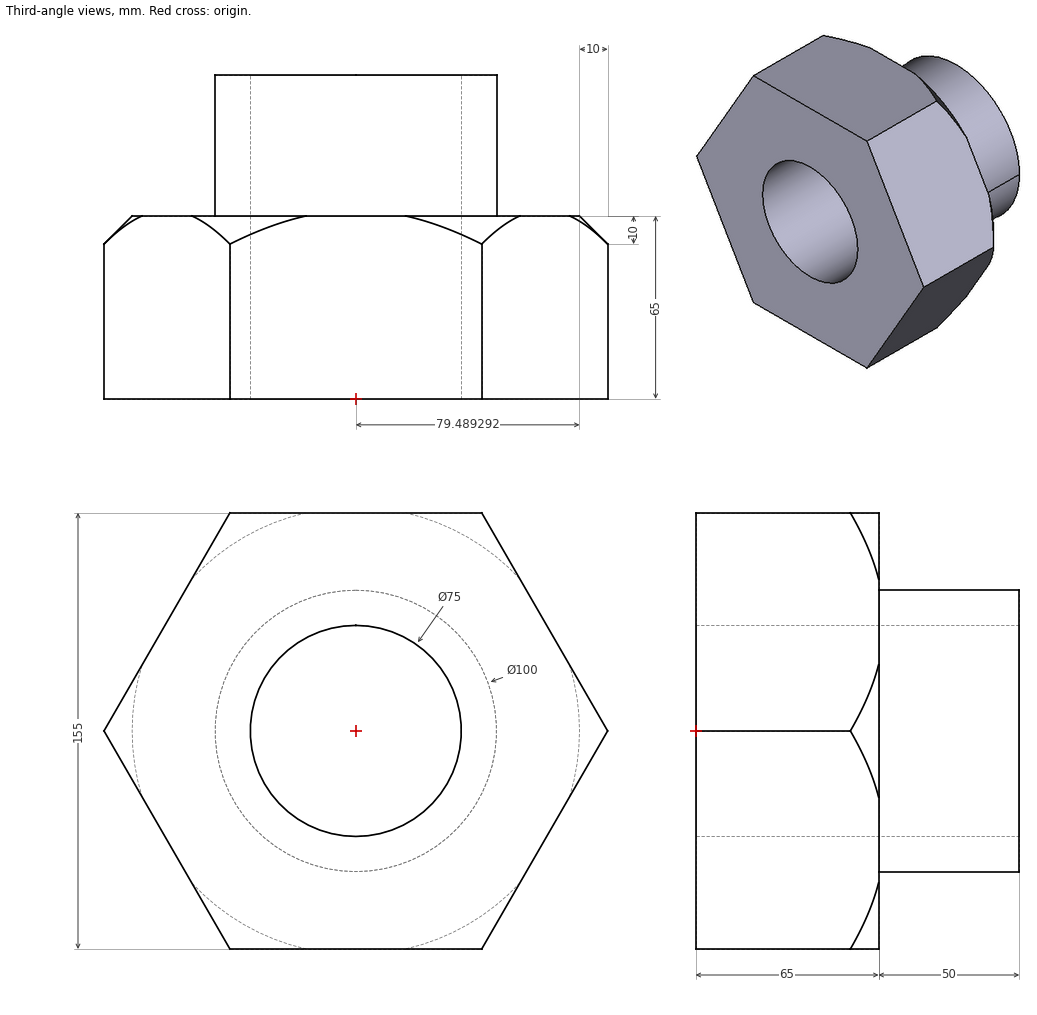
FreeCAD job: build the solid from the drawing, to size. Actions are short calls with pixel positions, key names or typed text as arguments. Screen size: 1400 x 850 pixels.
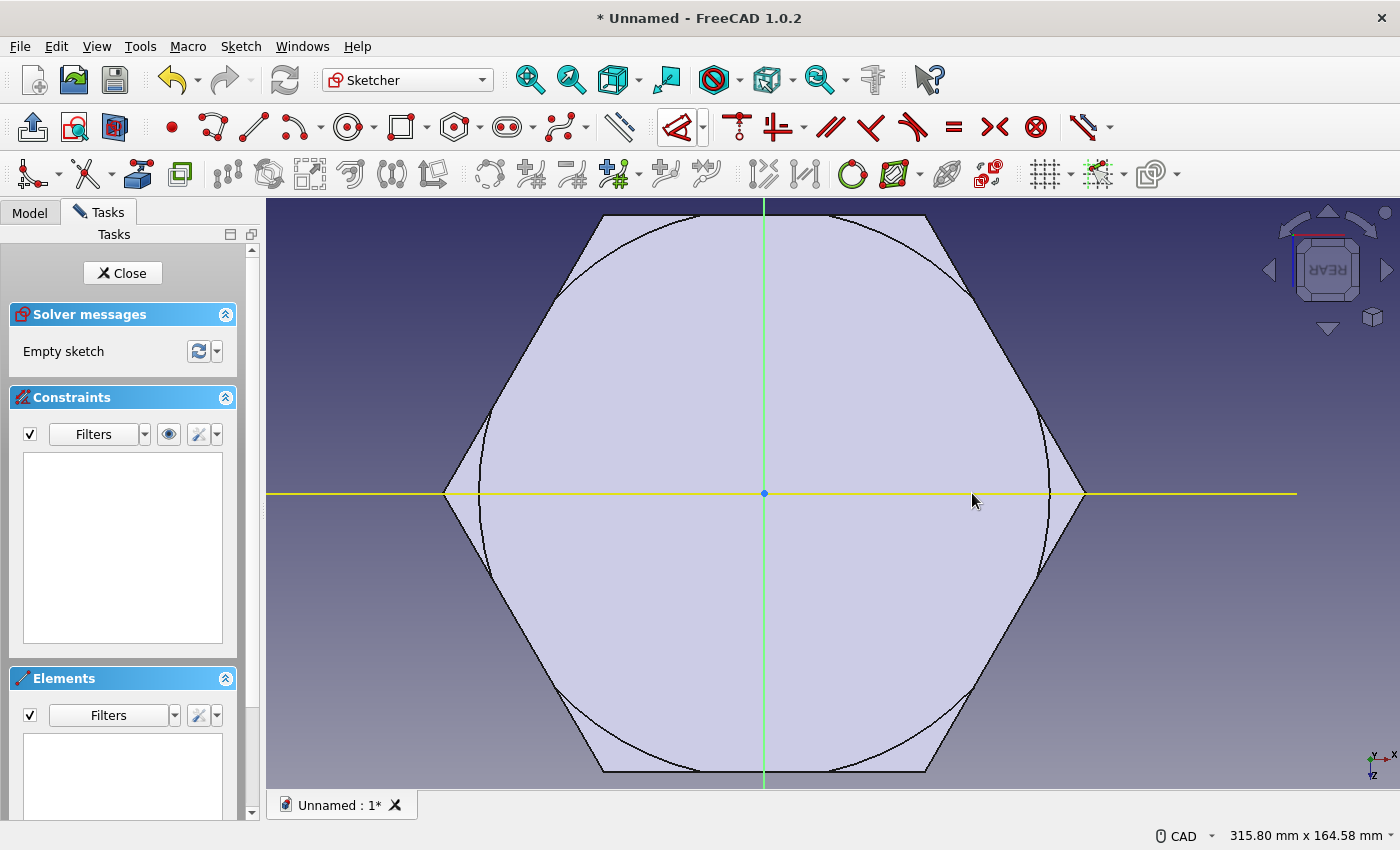
click(348, 128)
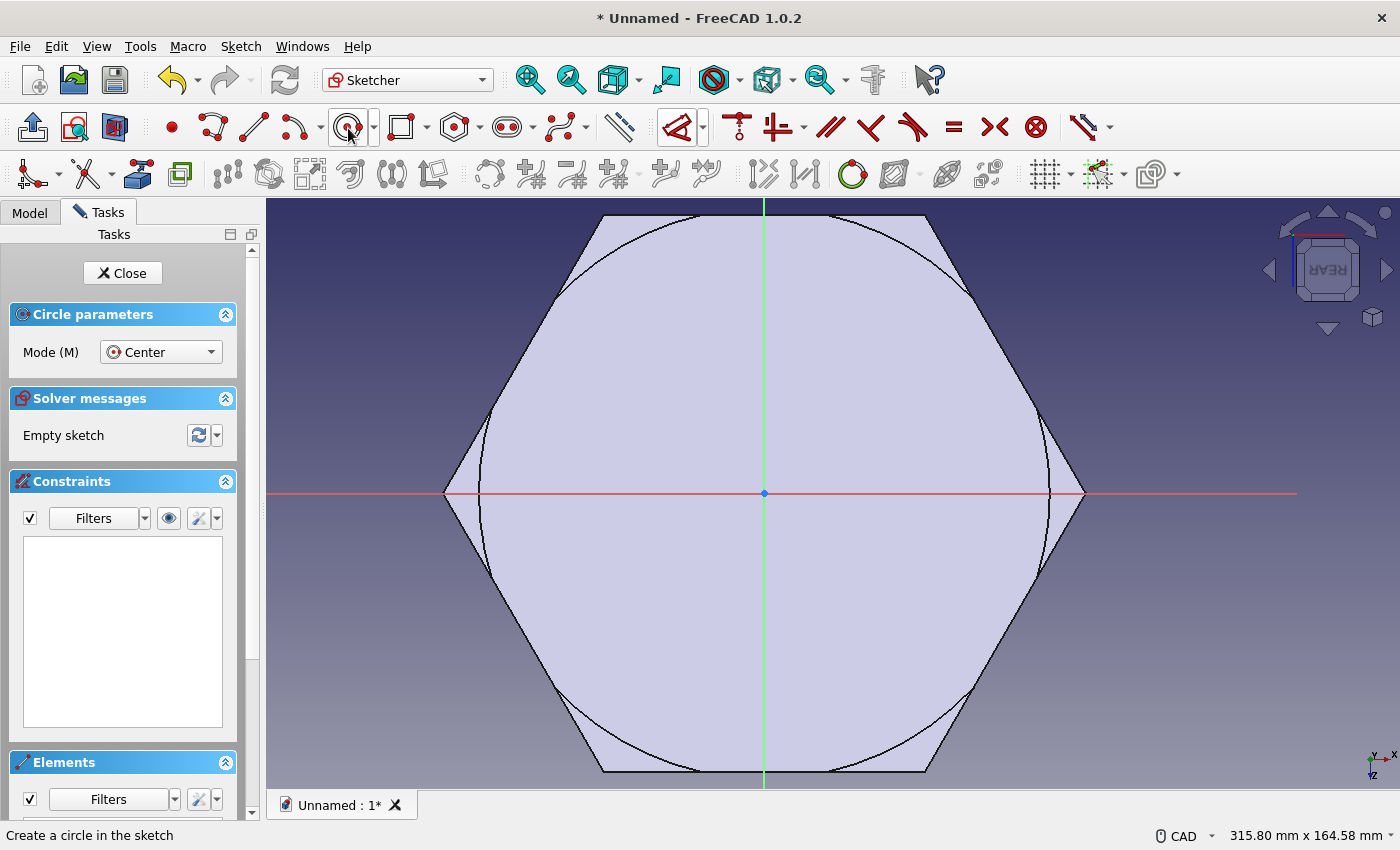
click(764, 493)
click(891, 367)
key(Escape)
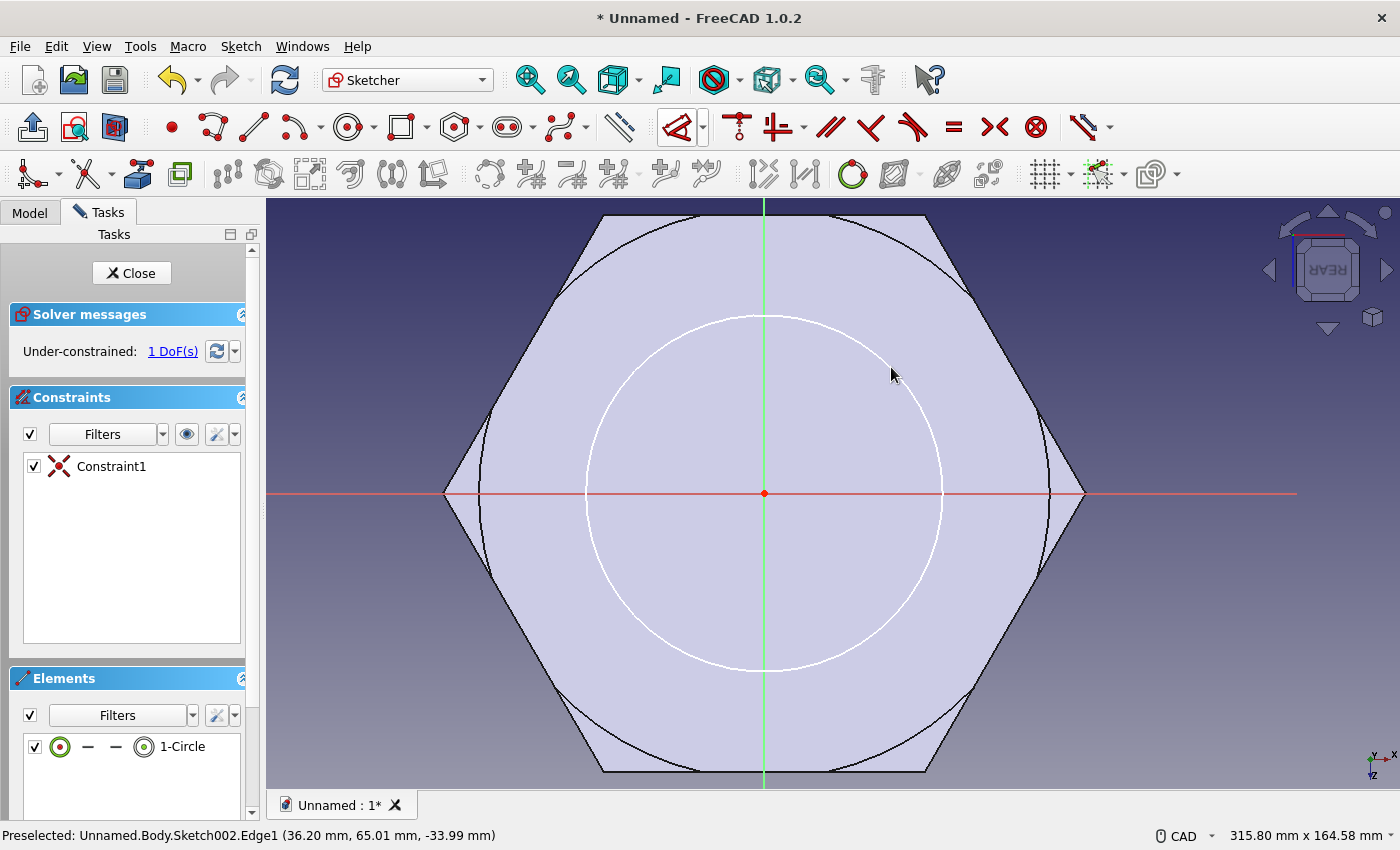
click(890, 367)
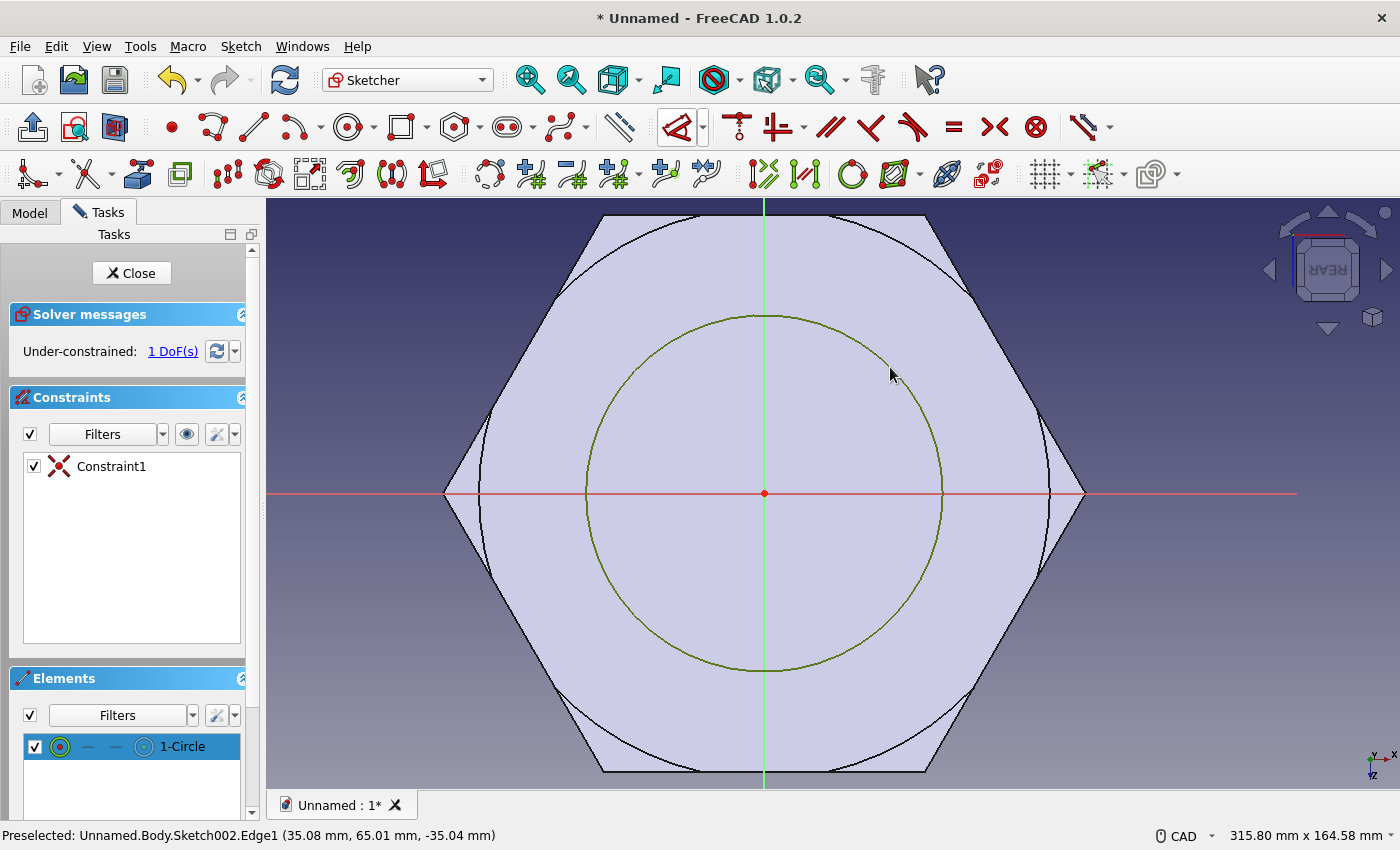
key(k)
key(o)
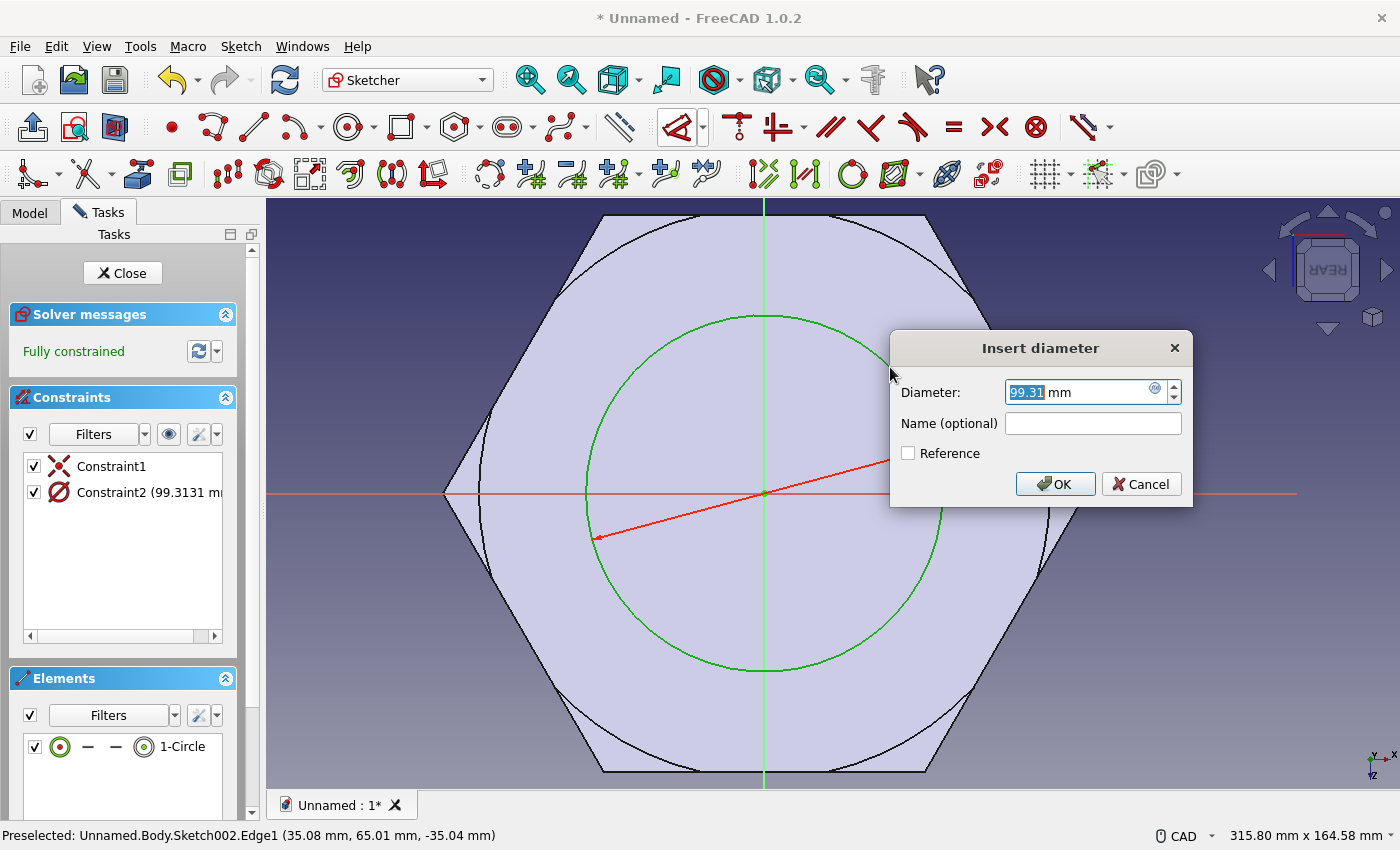
text(100)
key(Return)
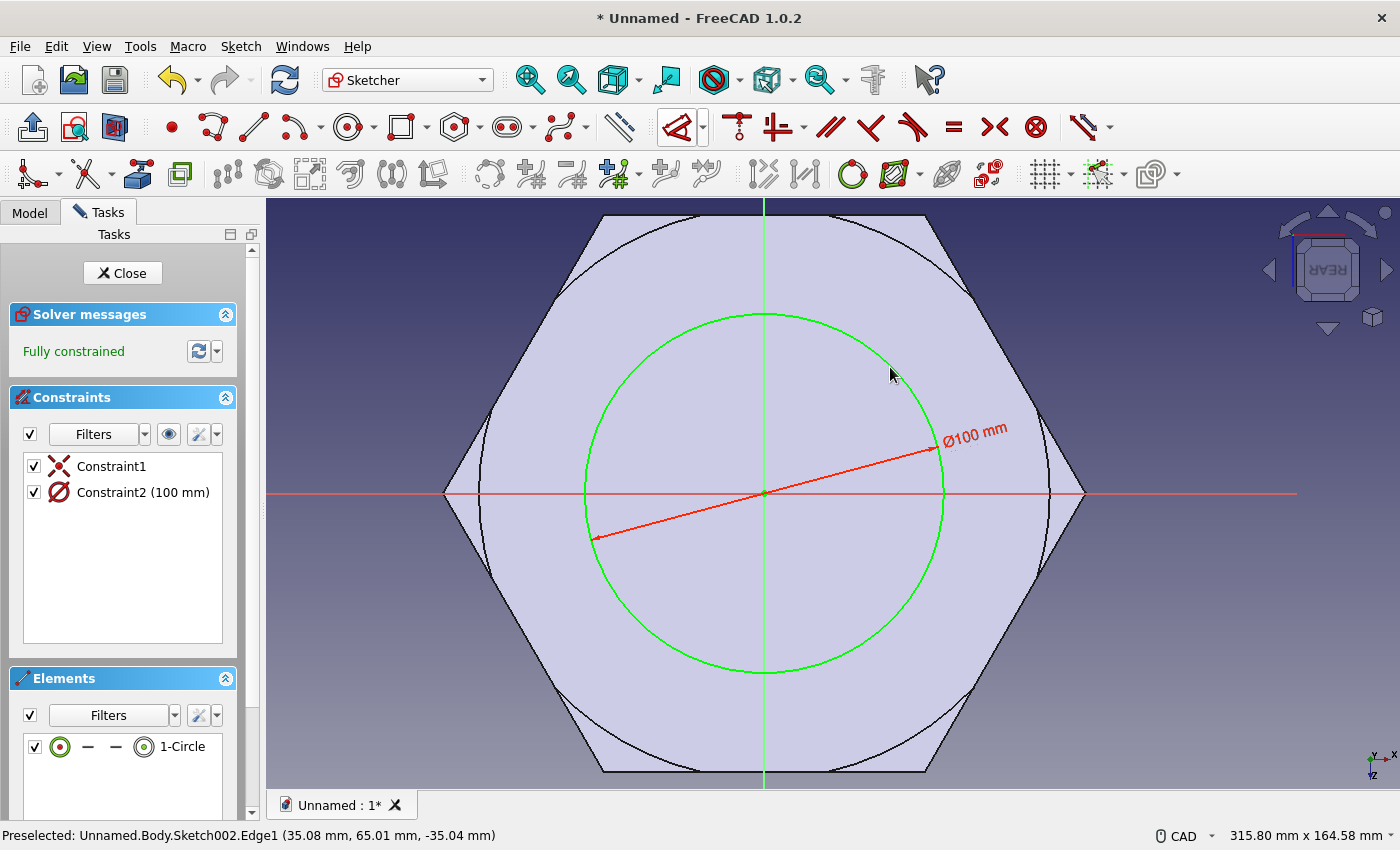
click(123, 273)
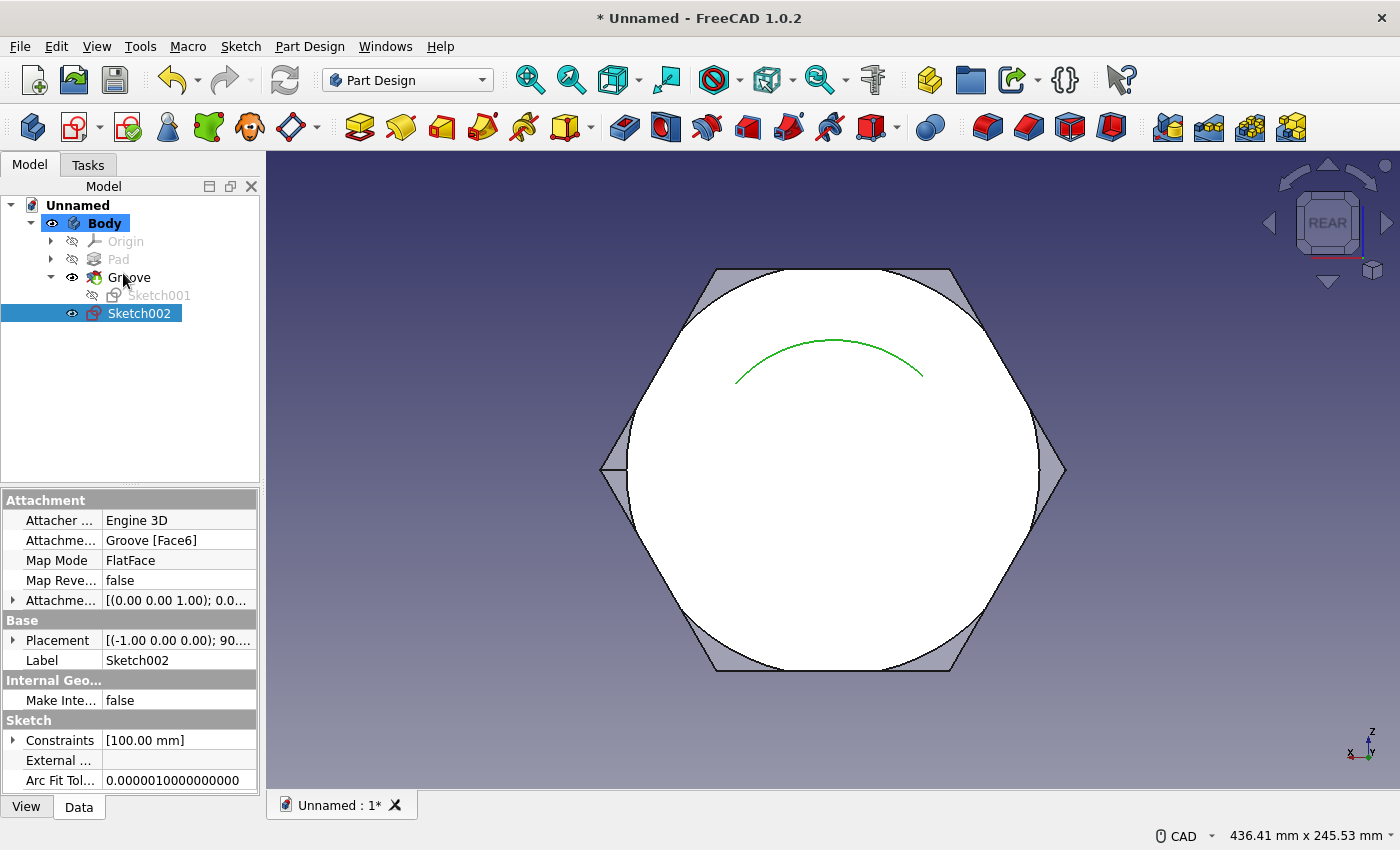
click(360, 128)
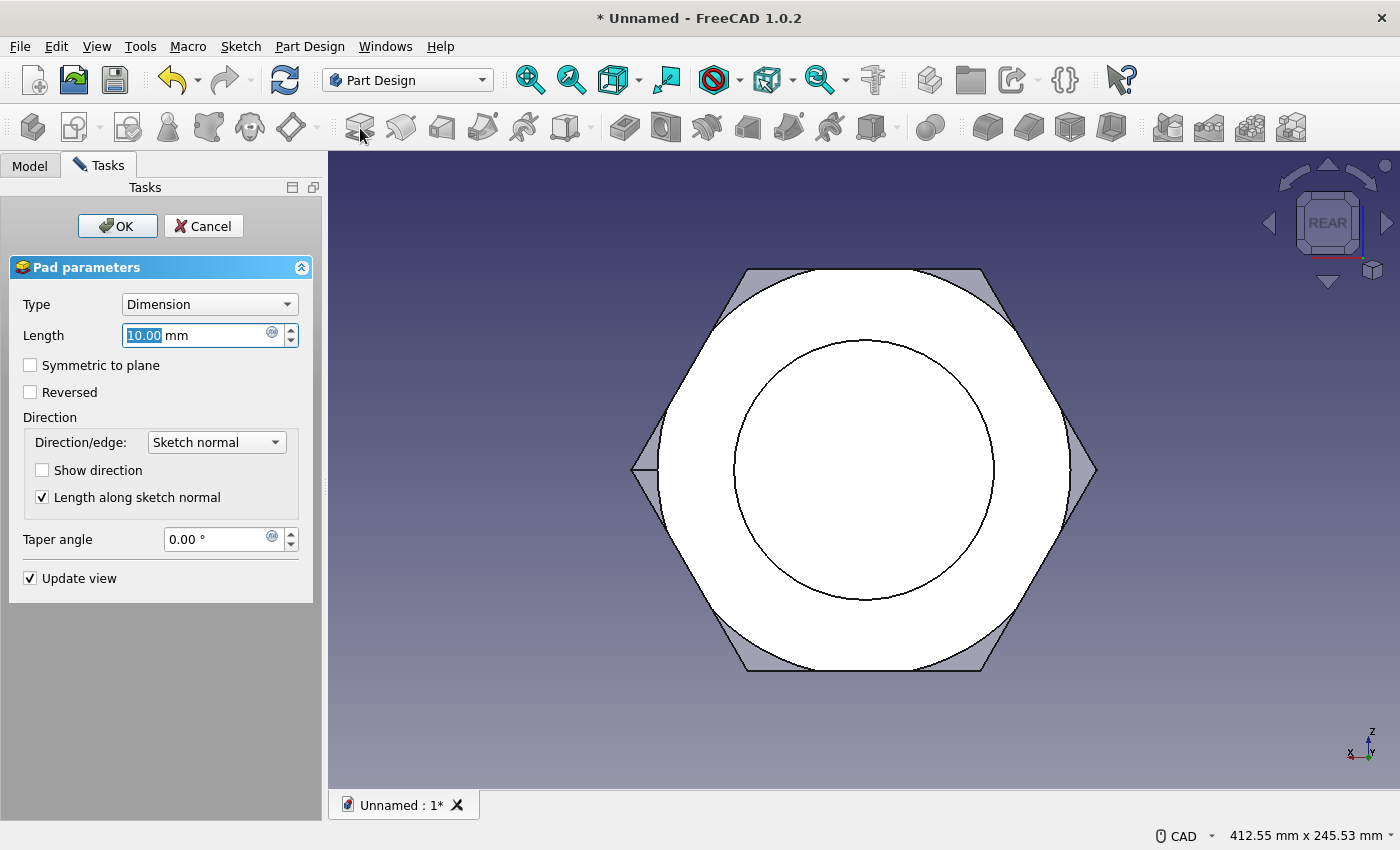
text(50)
key(Tab)